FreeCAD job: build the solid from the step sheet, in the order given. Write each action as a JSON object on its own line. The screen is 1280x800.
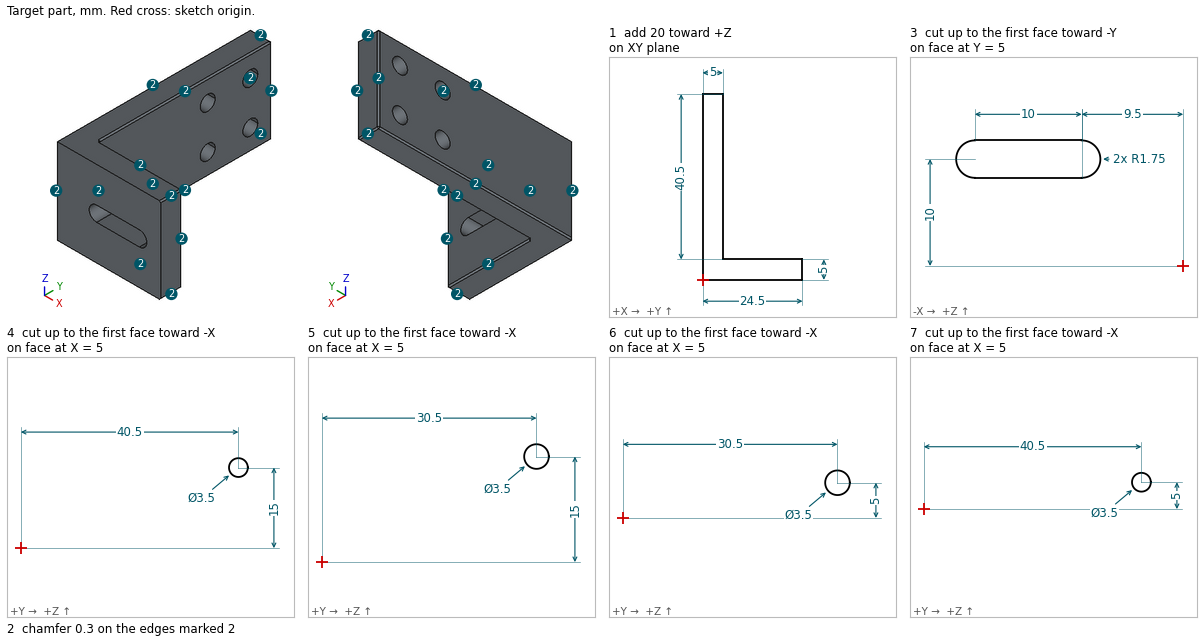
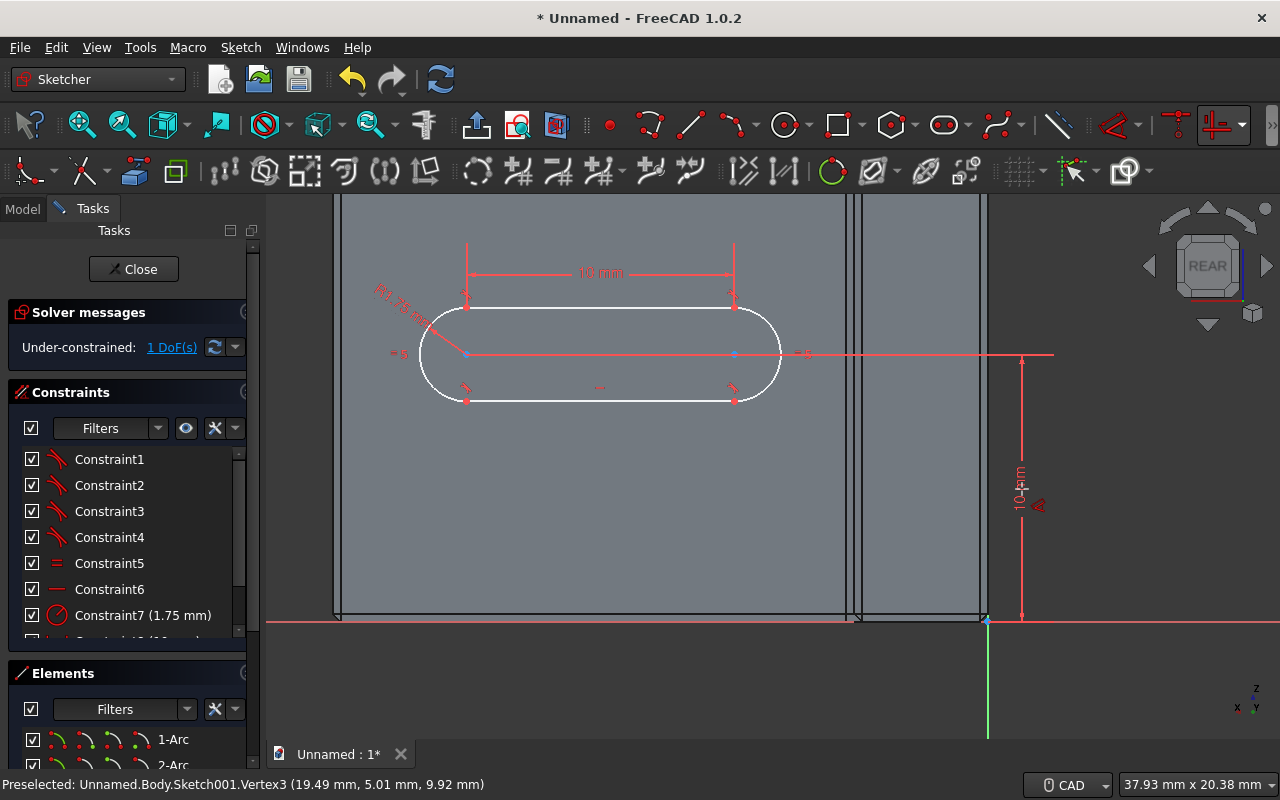
{"action": "left_click", "coordinate": [734, 401]}
{"action": "left_click", "coordinate": [861, 656]}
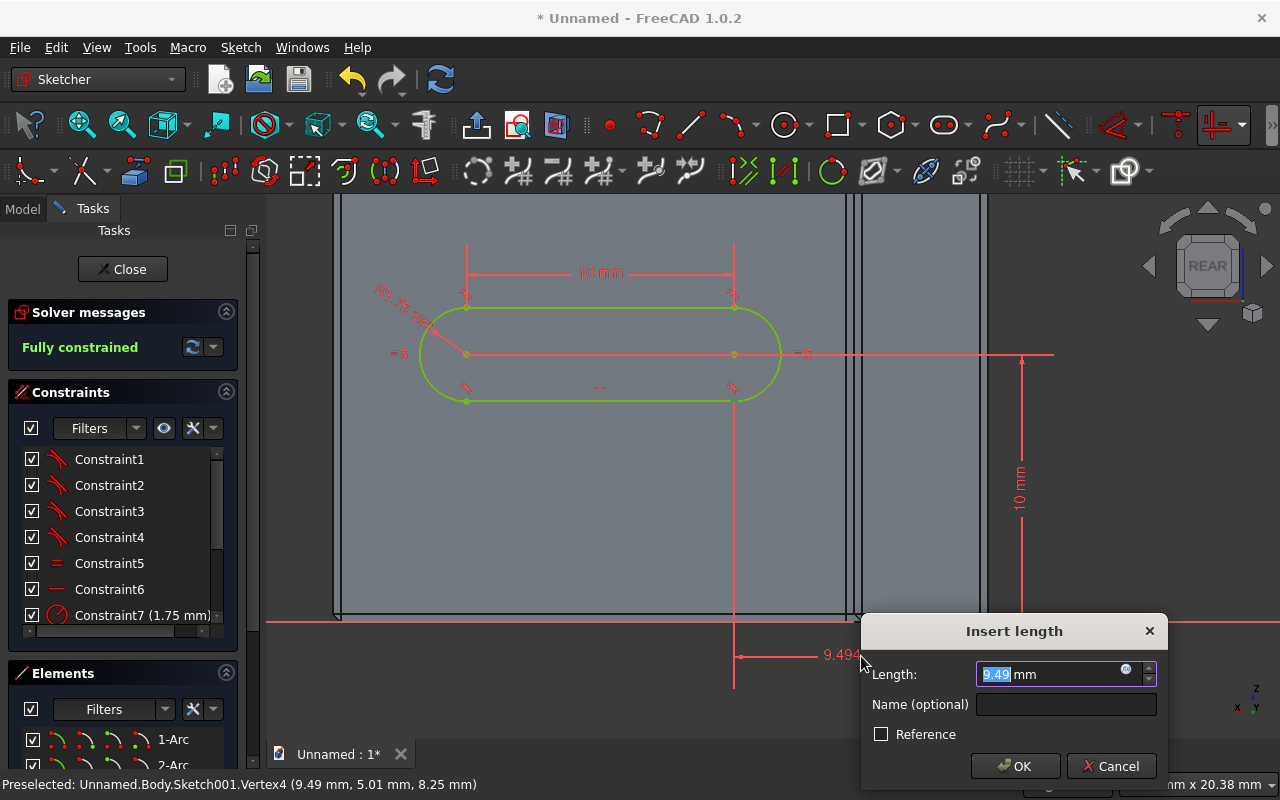
{"action": "type", "text": "9.5"}
{"action": "key", "text": "Return"}
{"action": "key", "text": "Escape"}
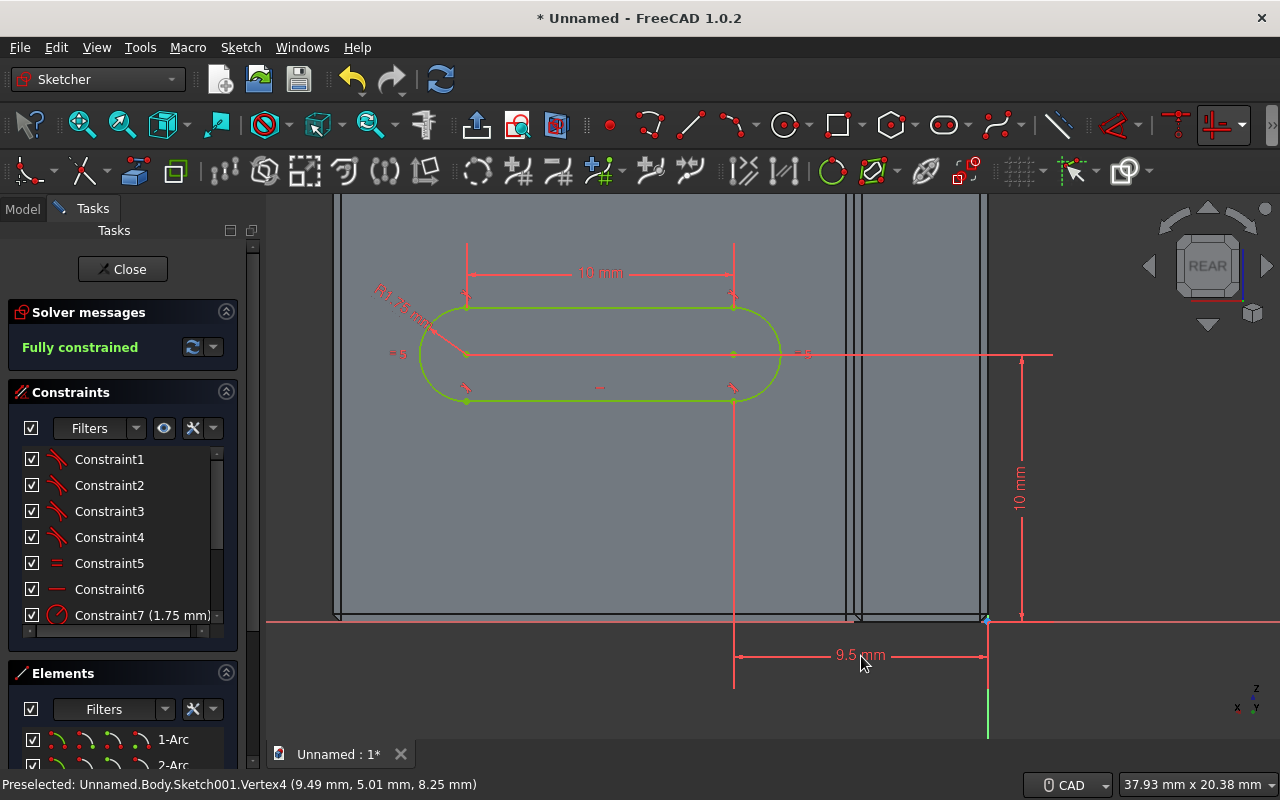
{"action": "left_click", "coordinate": [123, 269]}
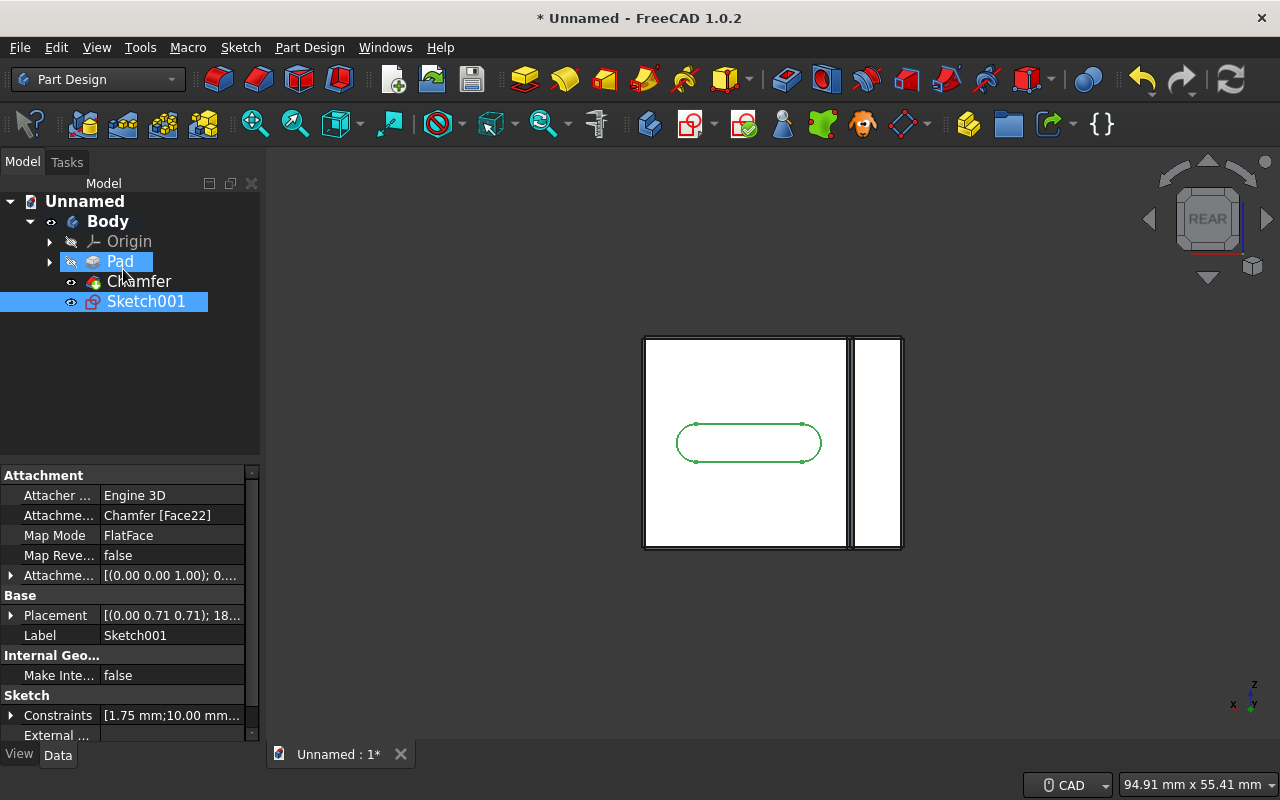
{"action": "left_click", "coordinate": [788, 80]}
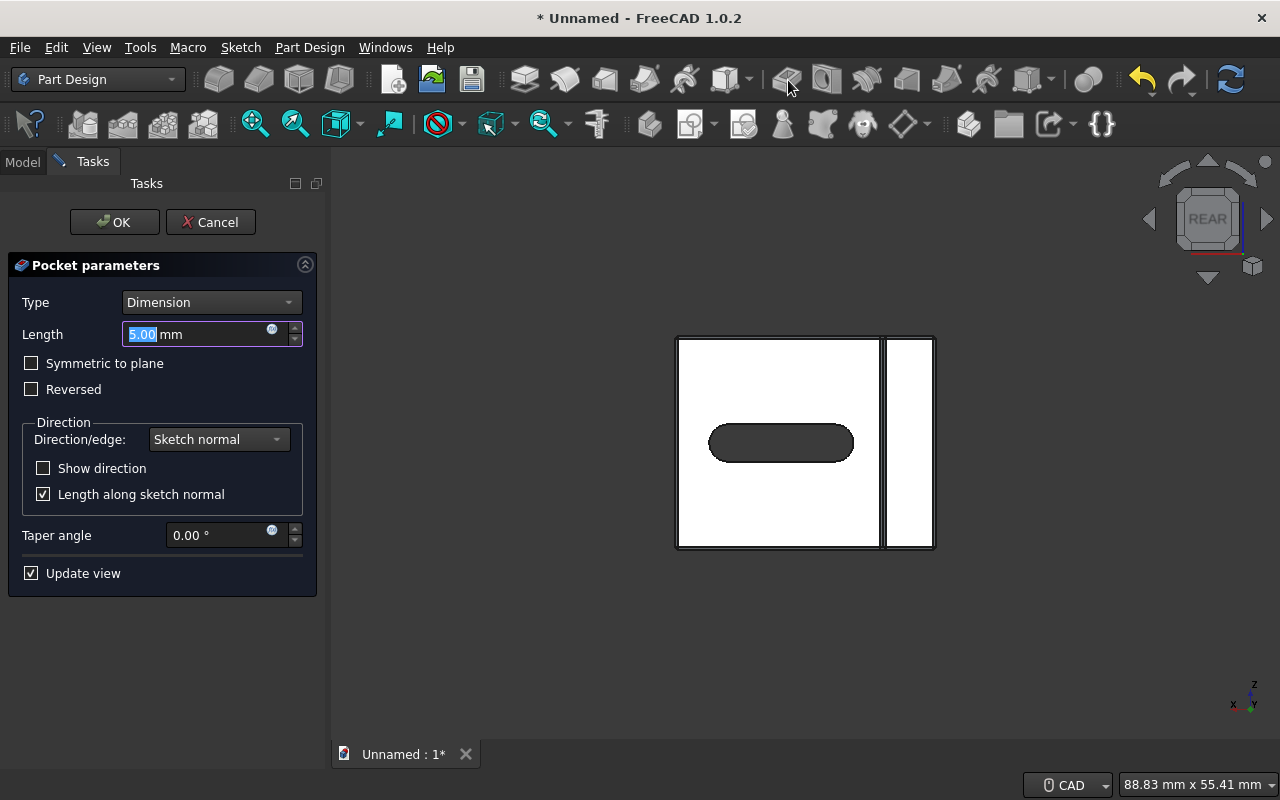
{"action": "left_click", "coordinate": [212, 302]}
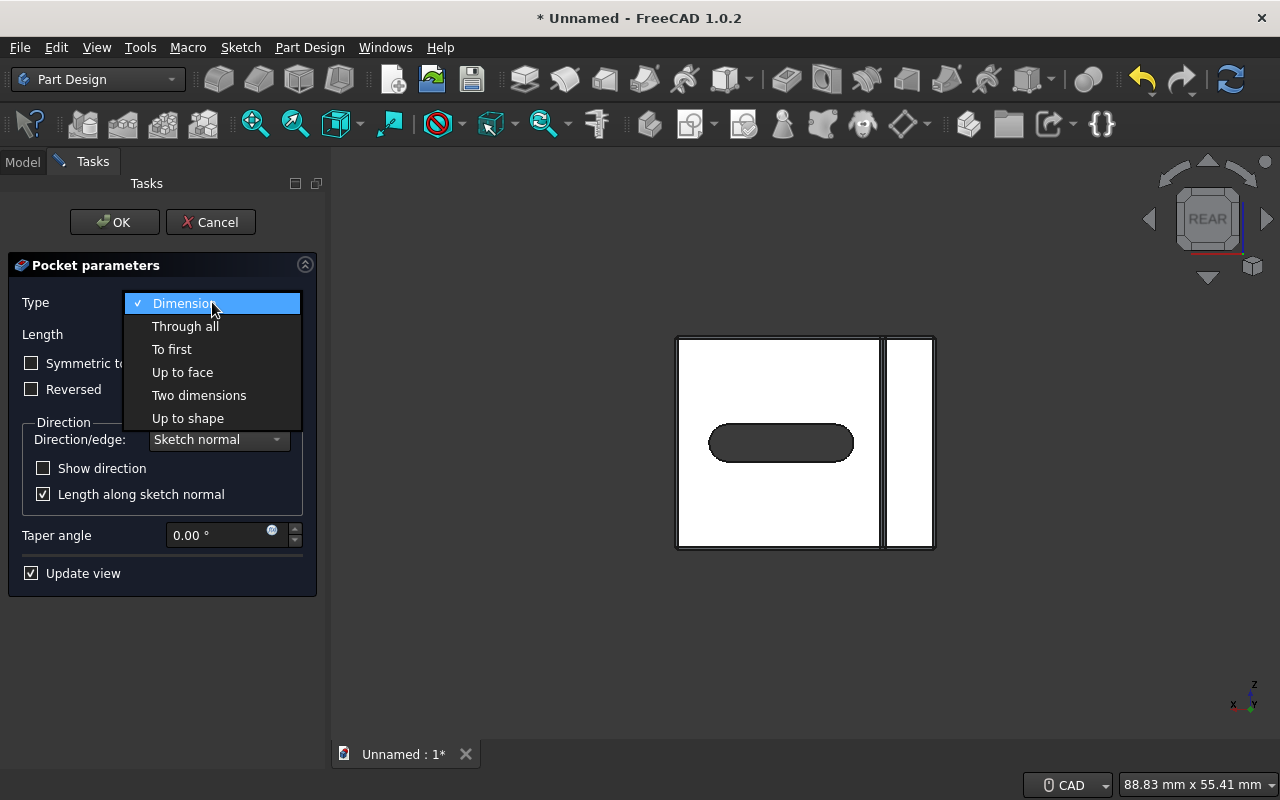
{"action": "left_click", "coordinate": [212, 350]}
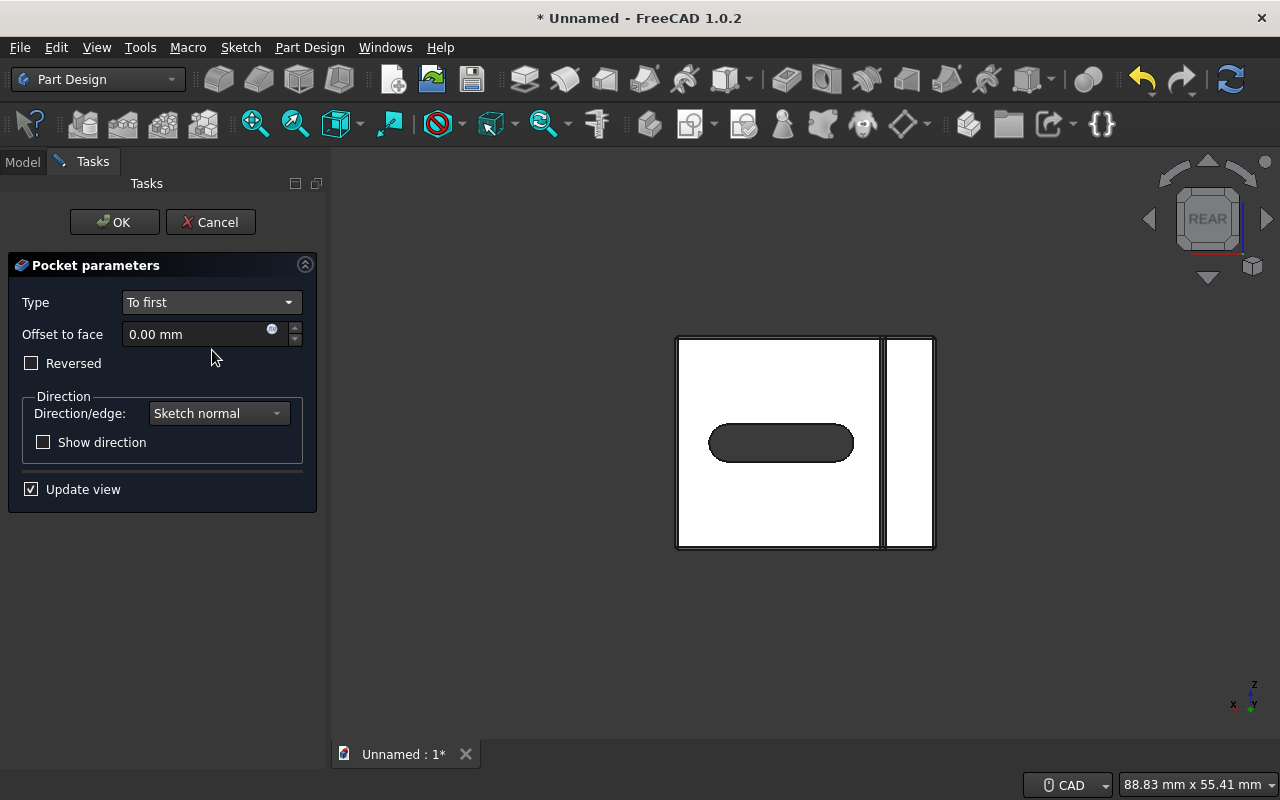
{"action": "left_click", "coordinate": [115, 222]}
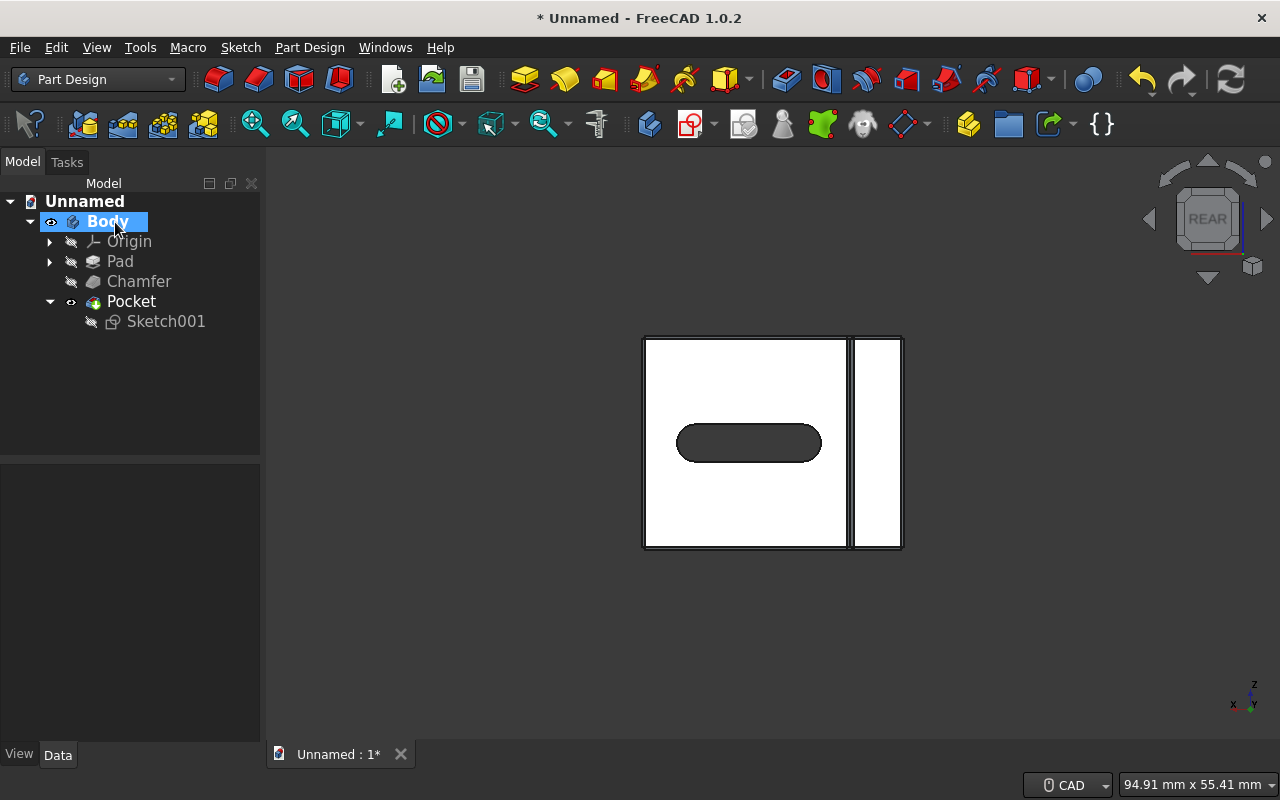
{"action": "key", "text": "v f"}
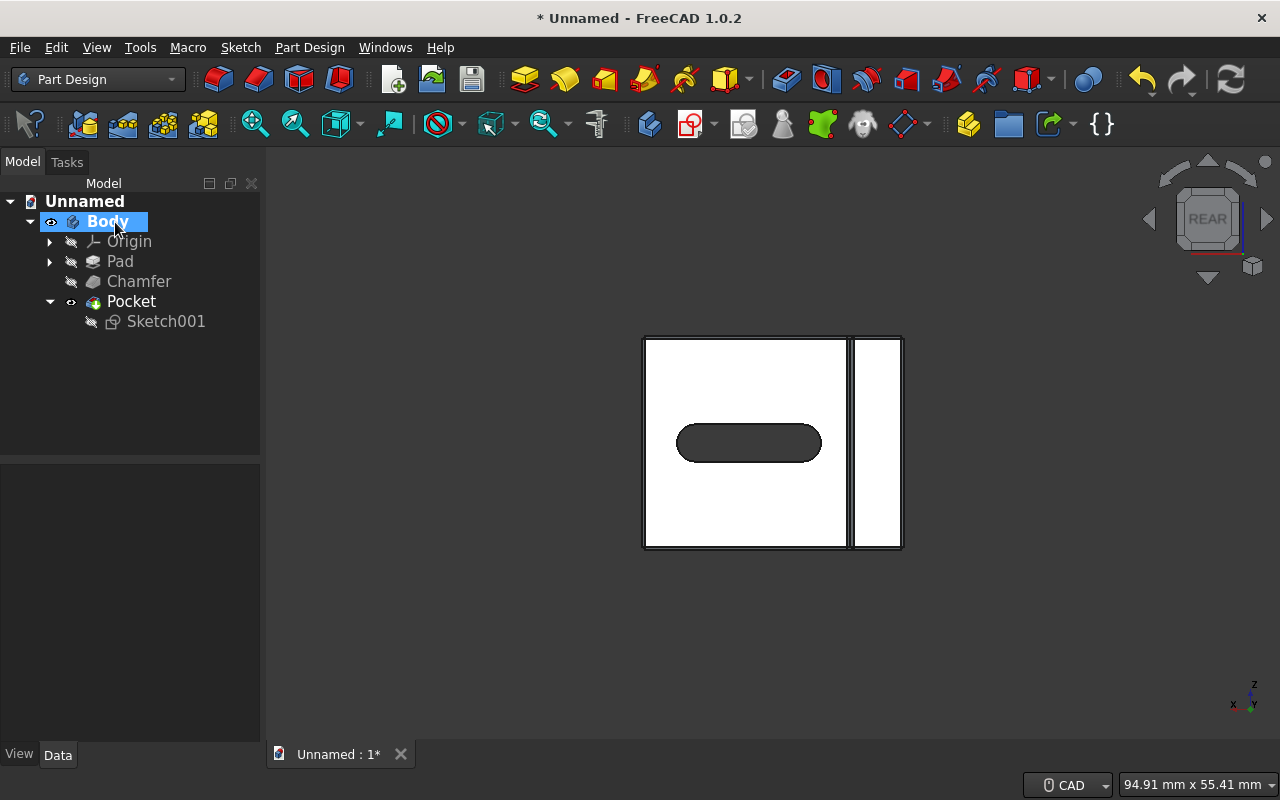
{"action": "key", "text": "0"}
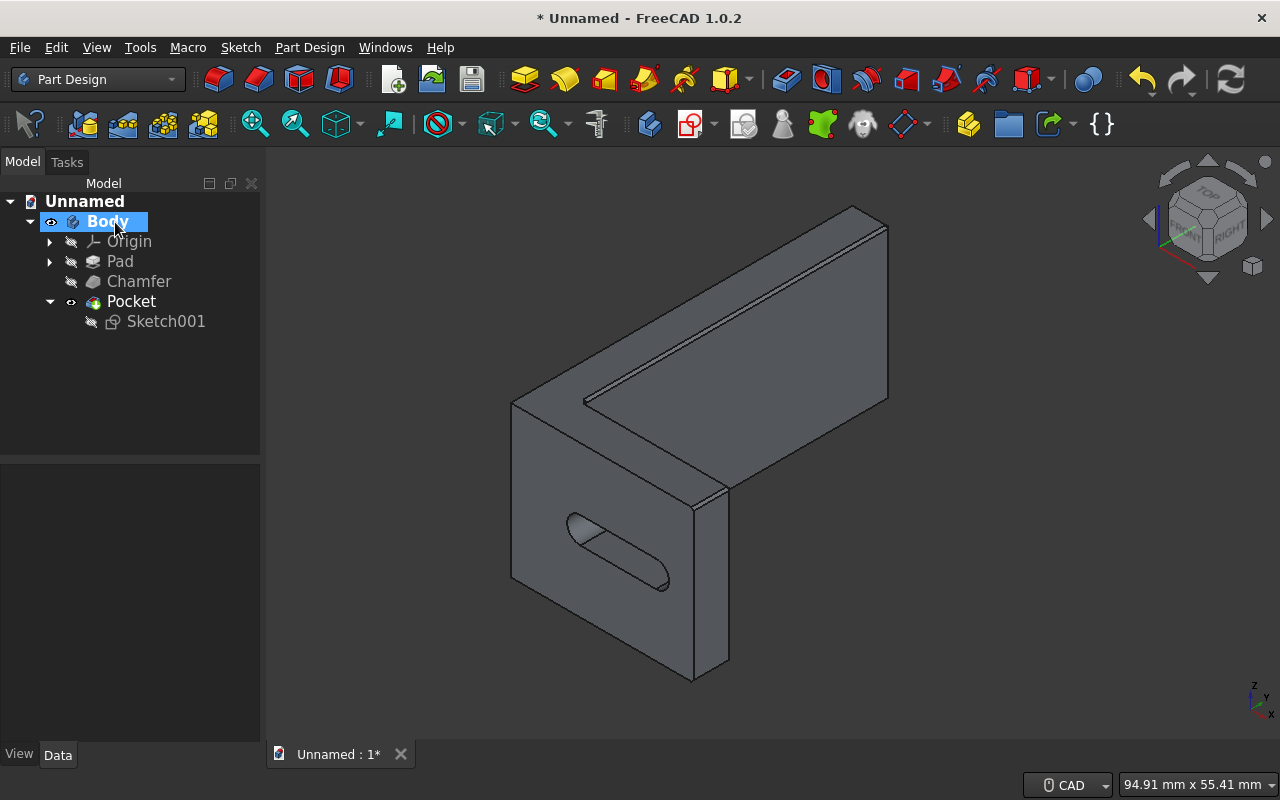
{"action": "left_click", "coordinate": [780, 375]}